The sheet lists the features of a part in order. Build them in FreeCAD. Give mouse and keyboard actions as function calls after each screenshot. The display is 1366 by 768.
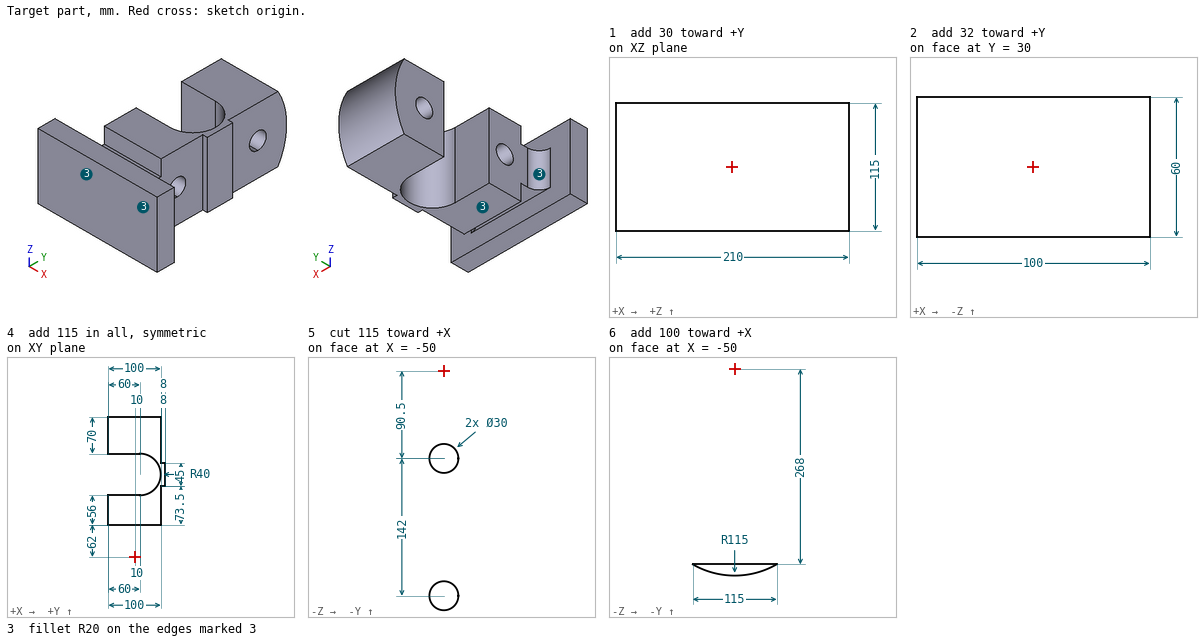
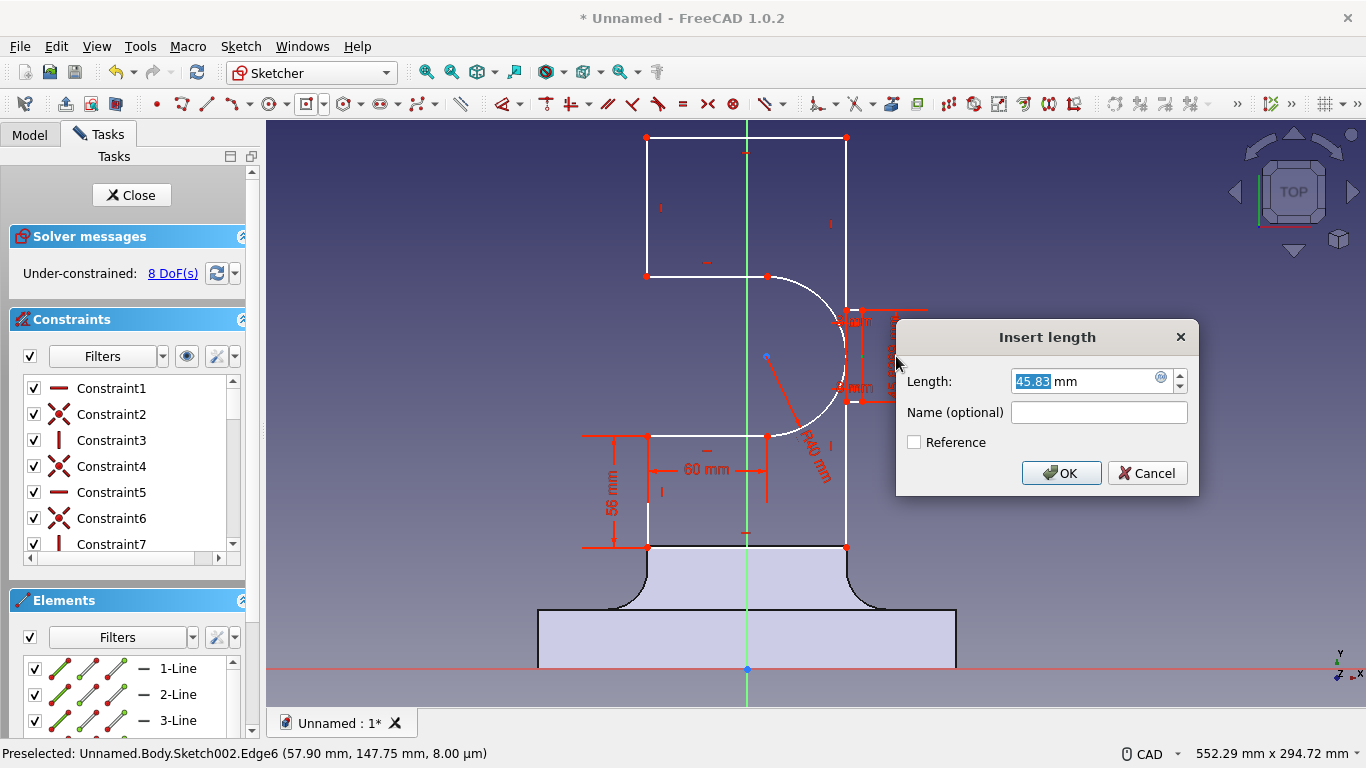
text(45)
key(Return)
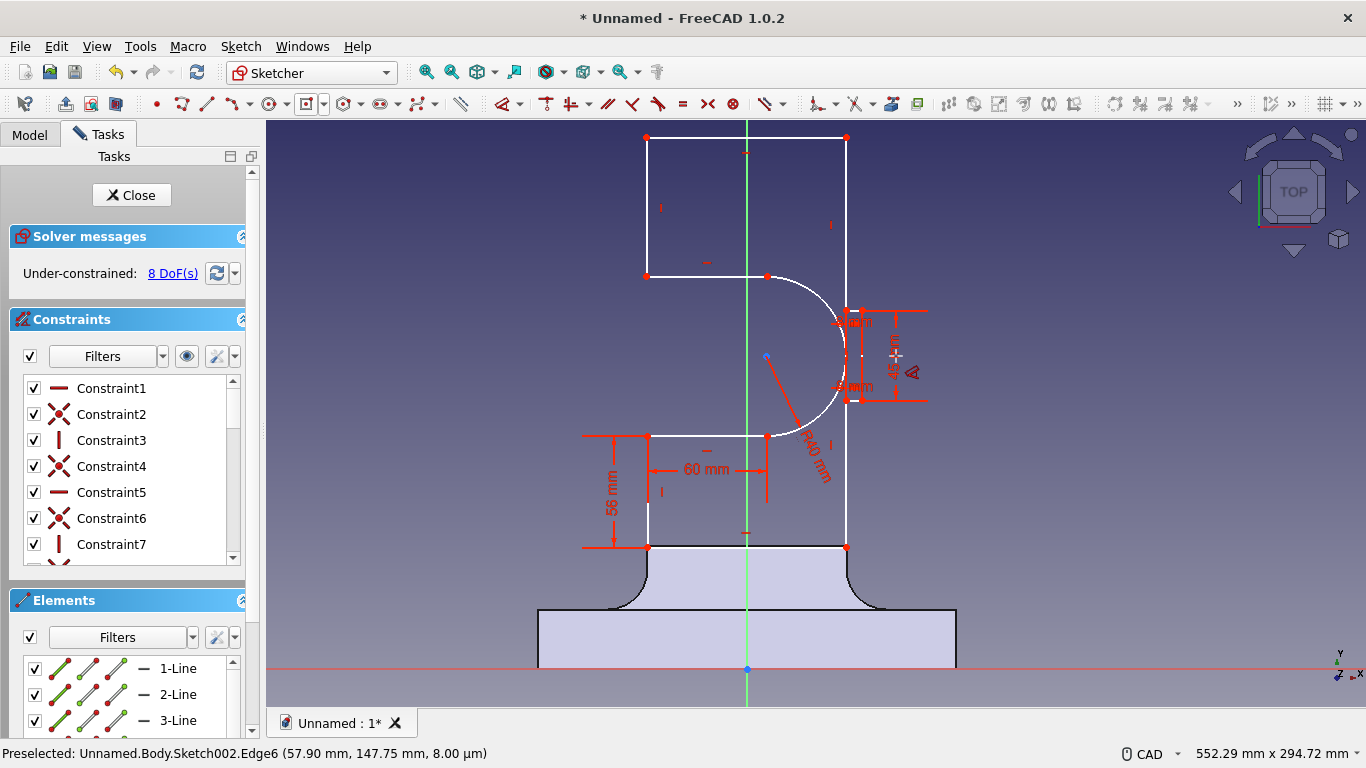
click(647, 179)
click(613, 212)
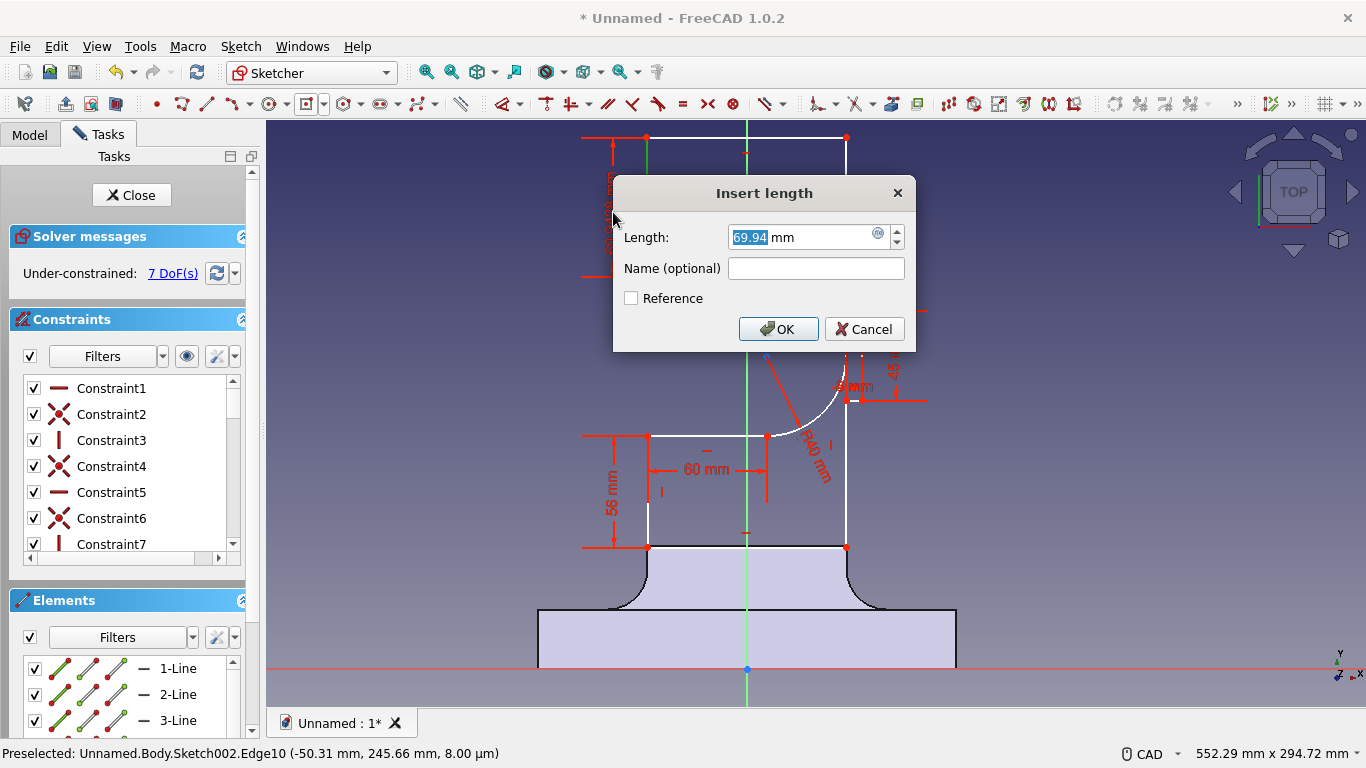
text(70)
key(Return)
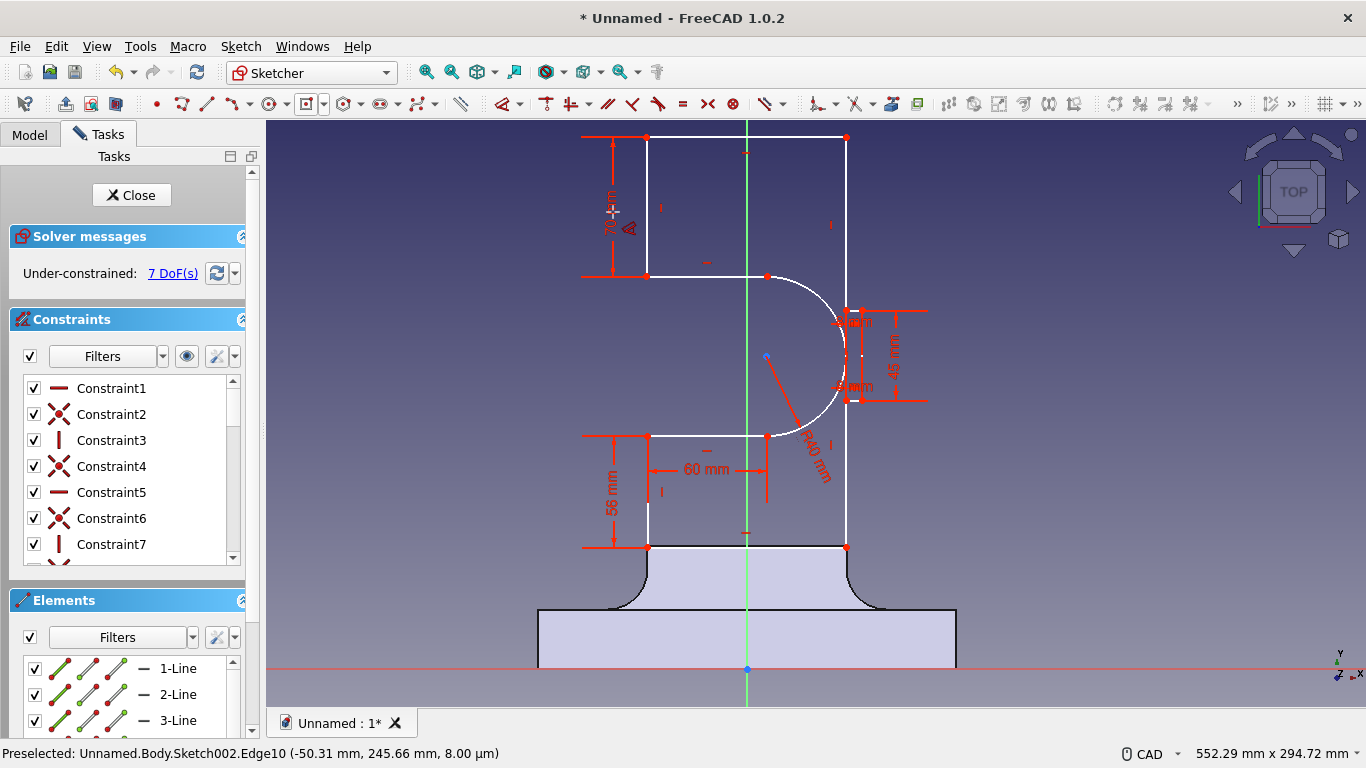
click(683, 277)
click(707, 243)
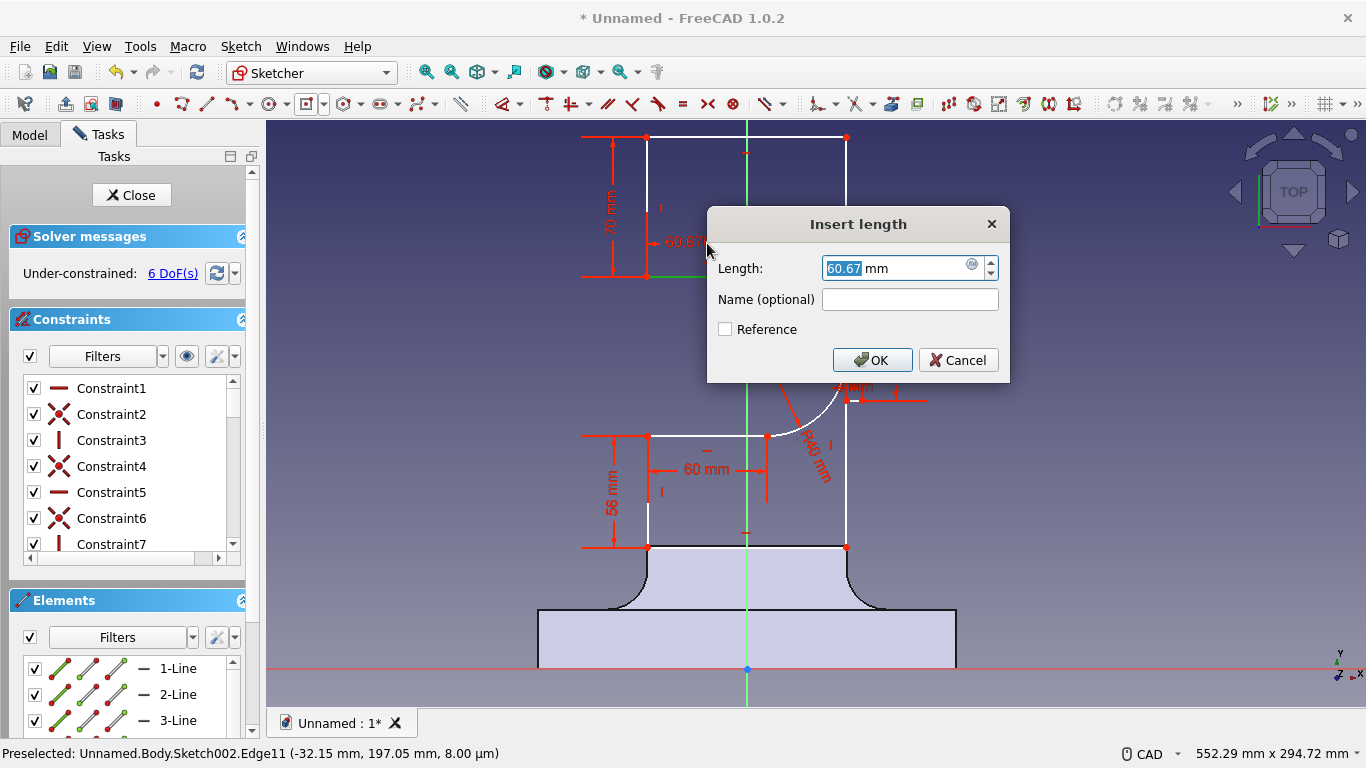
text(60)
key(Return)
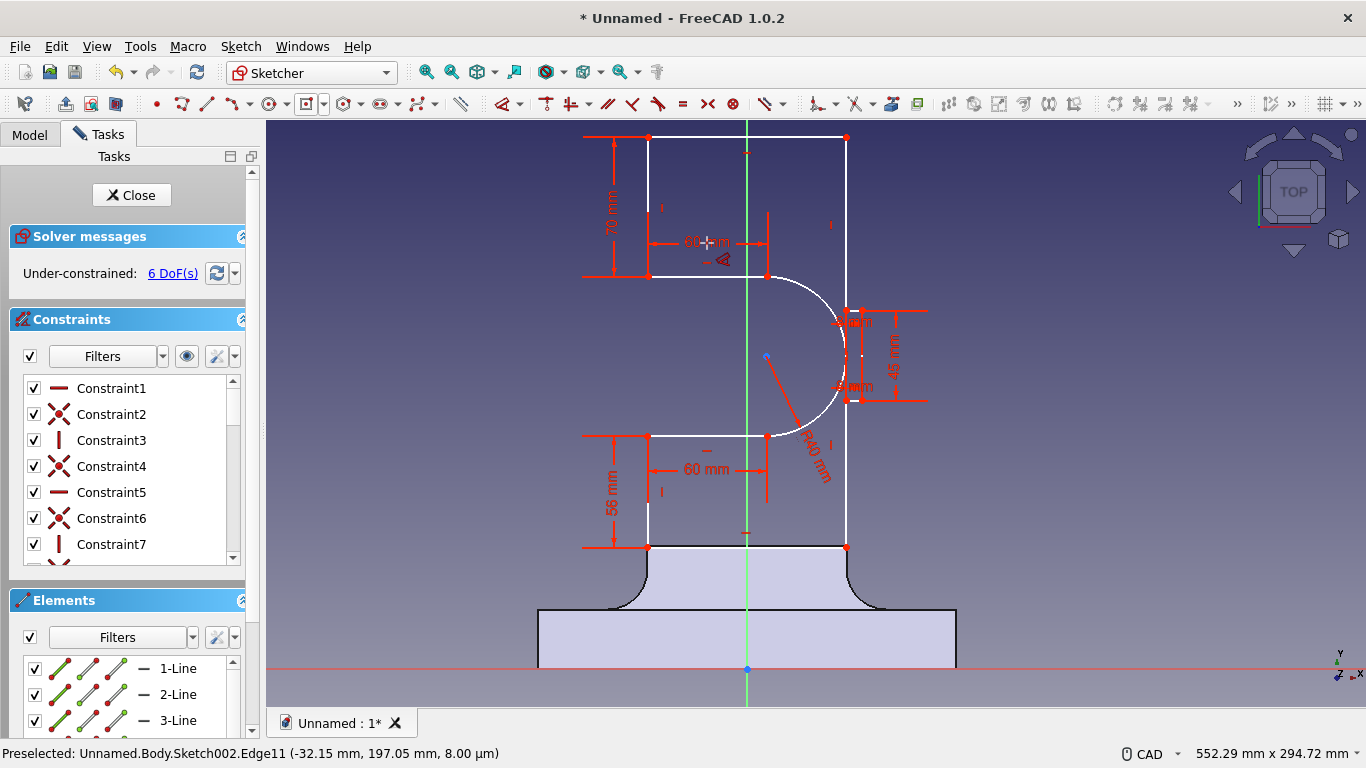
click(707, 548)
click(701, 582)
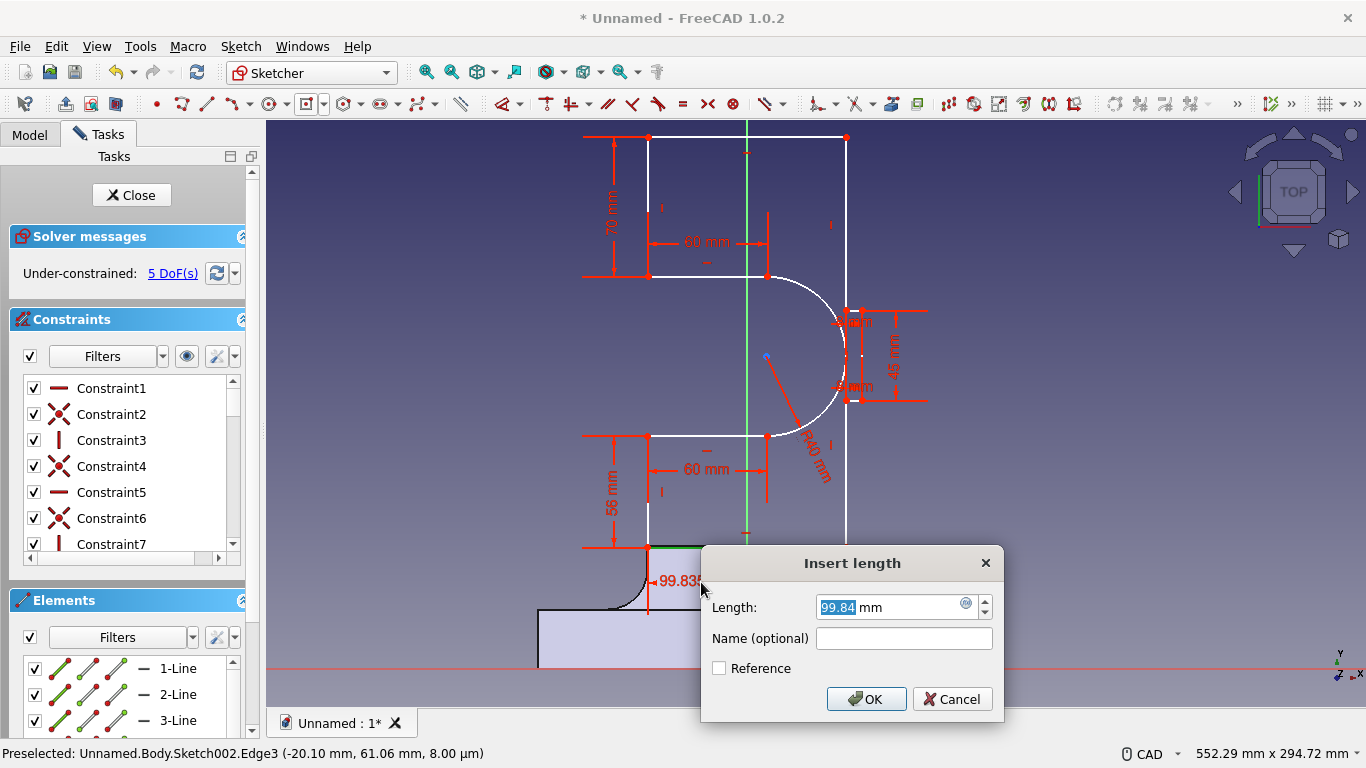
text(100)
key(Return)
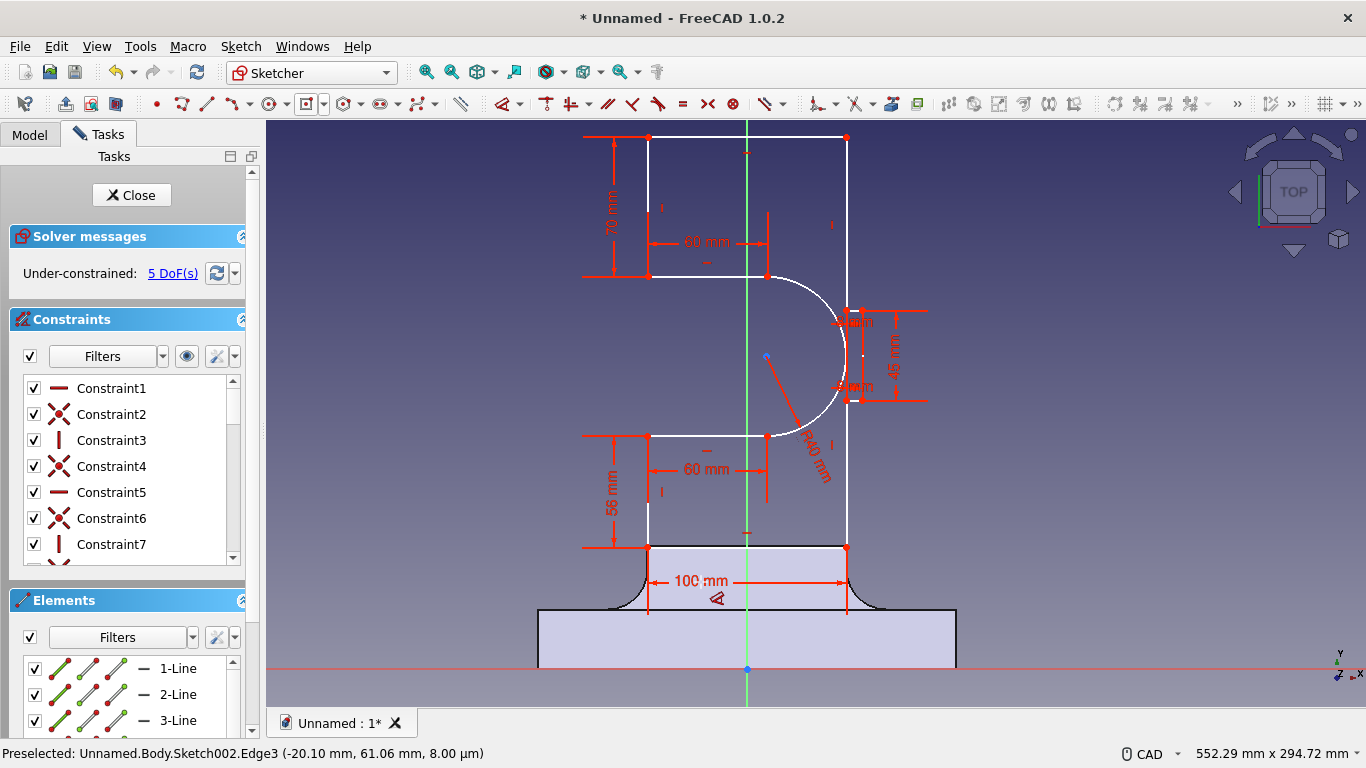
scroll(732, 436, down, 2)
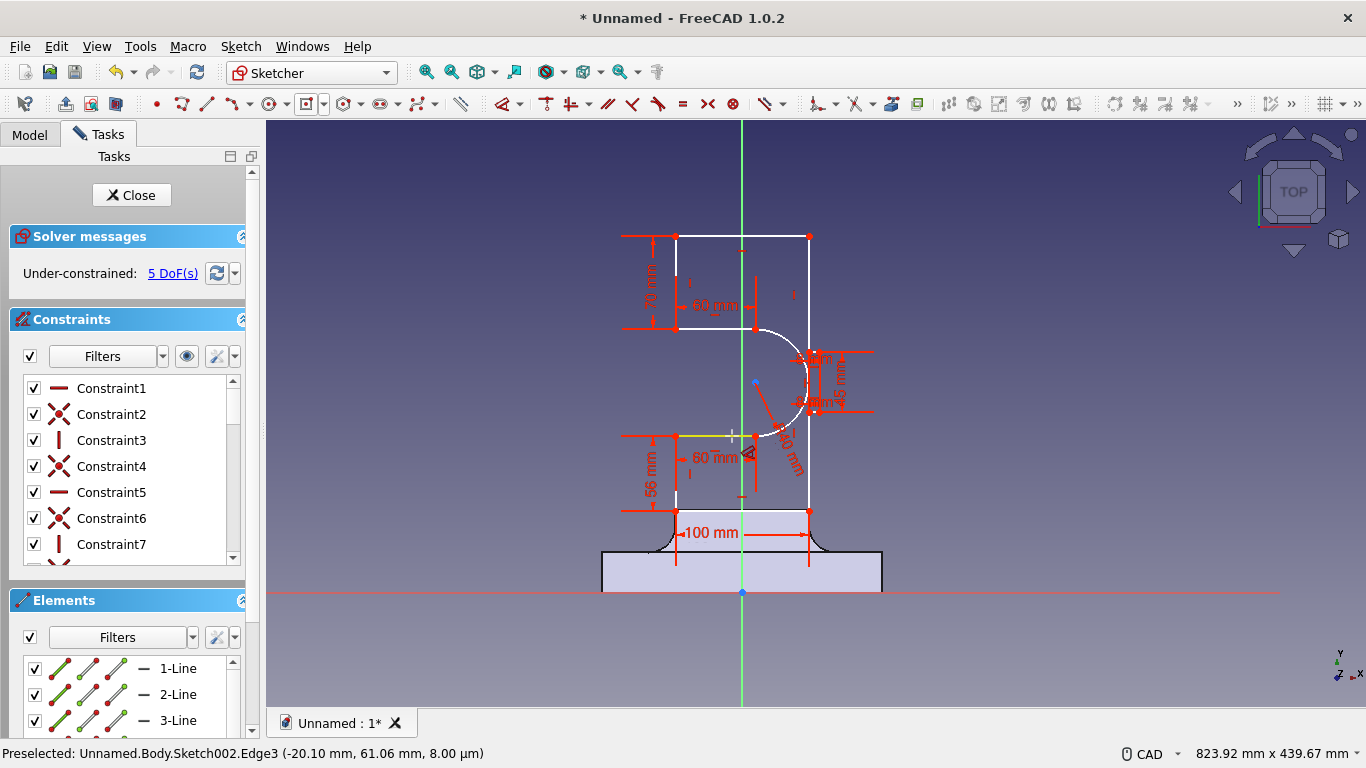
click(769, 236)
click(712, 202)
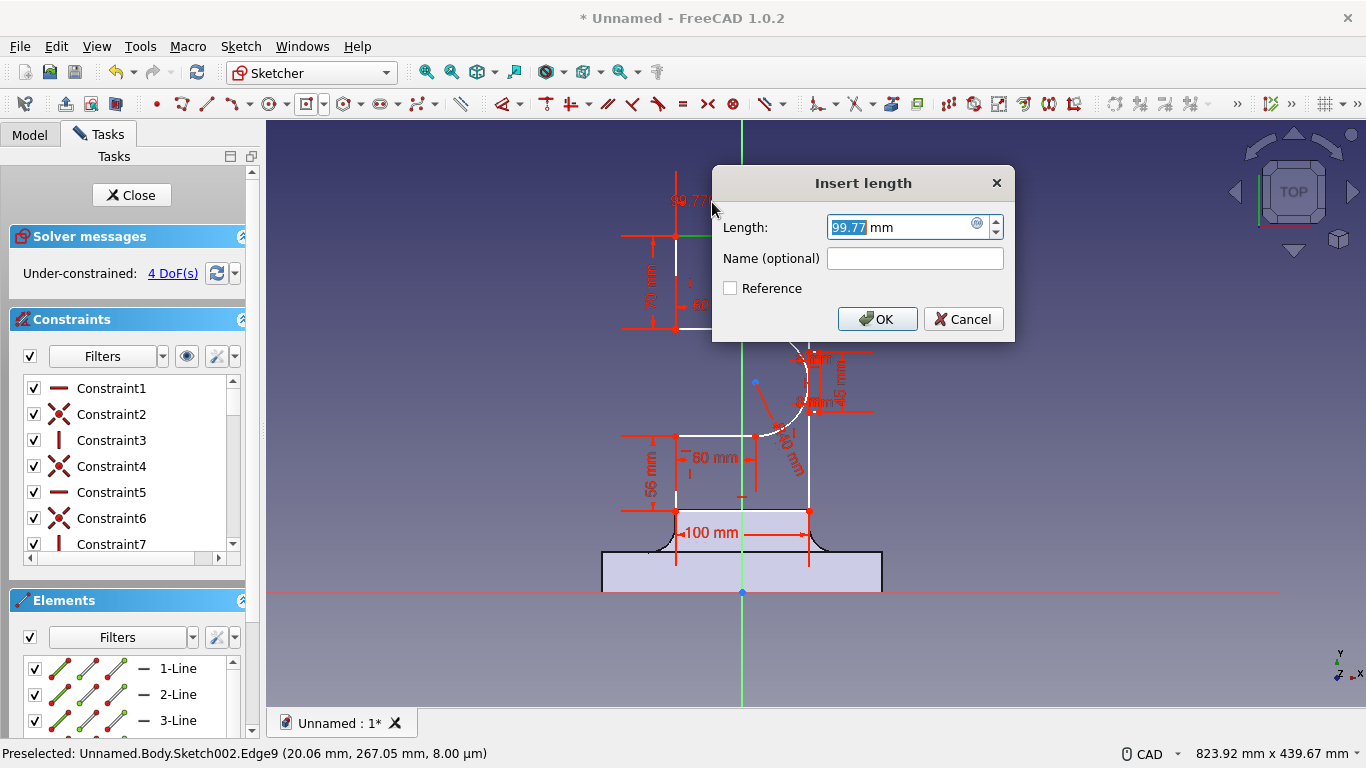
text(100)
key(Return)